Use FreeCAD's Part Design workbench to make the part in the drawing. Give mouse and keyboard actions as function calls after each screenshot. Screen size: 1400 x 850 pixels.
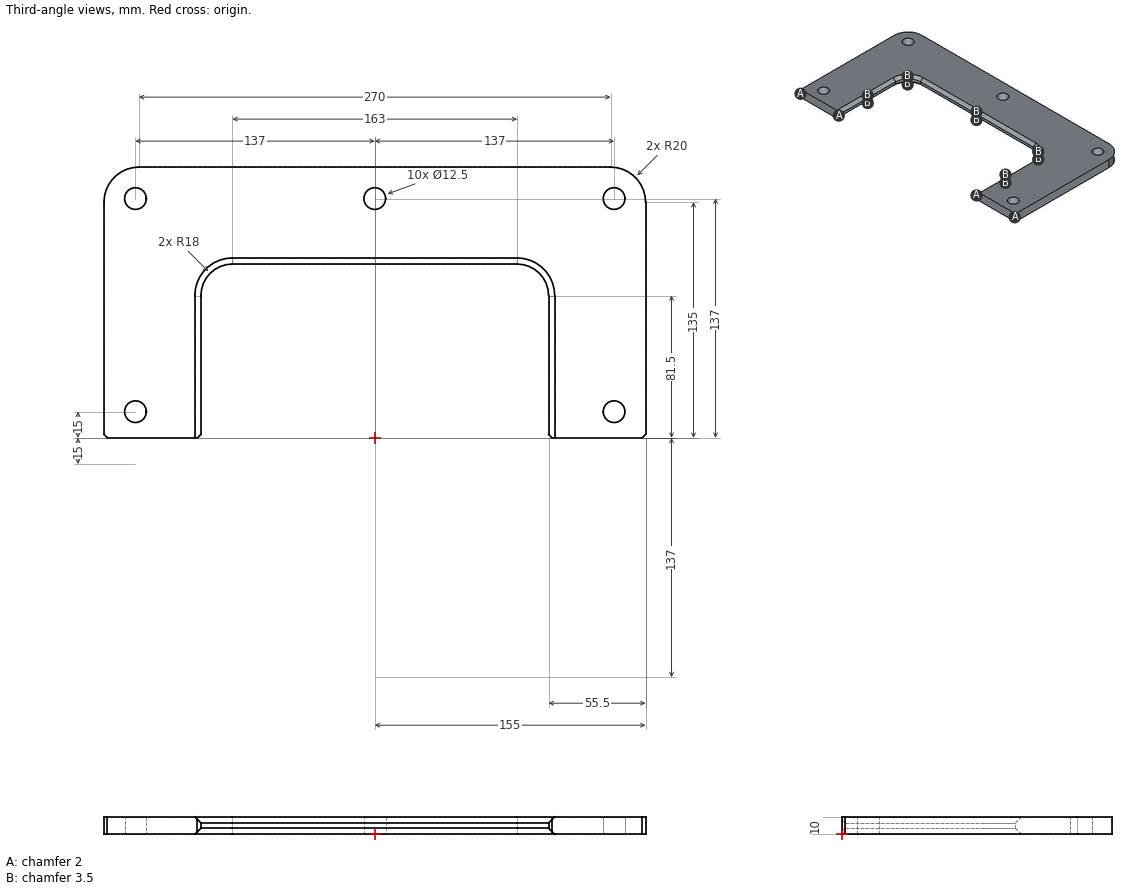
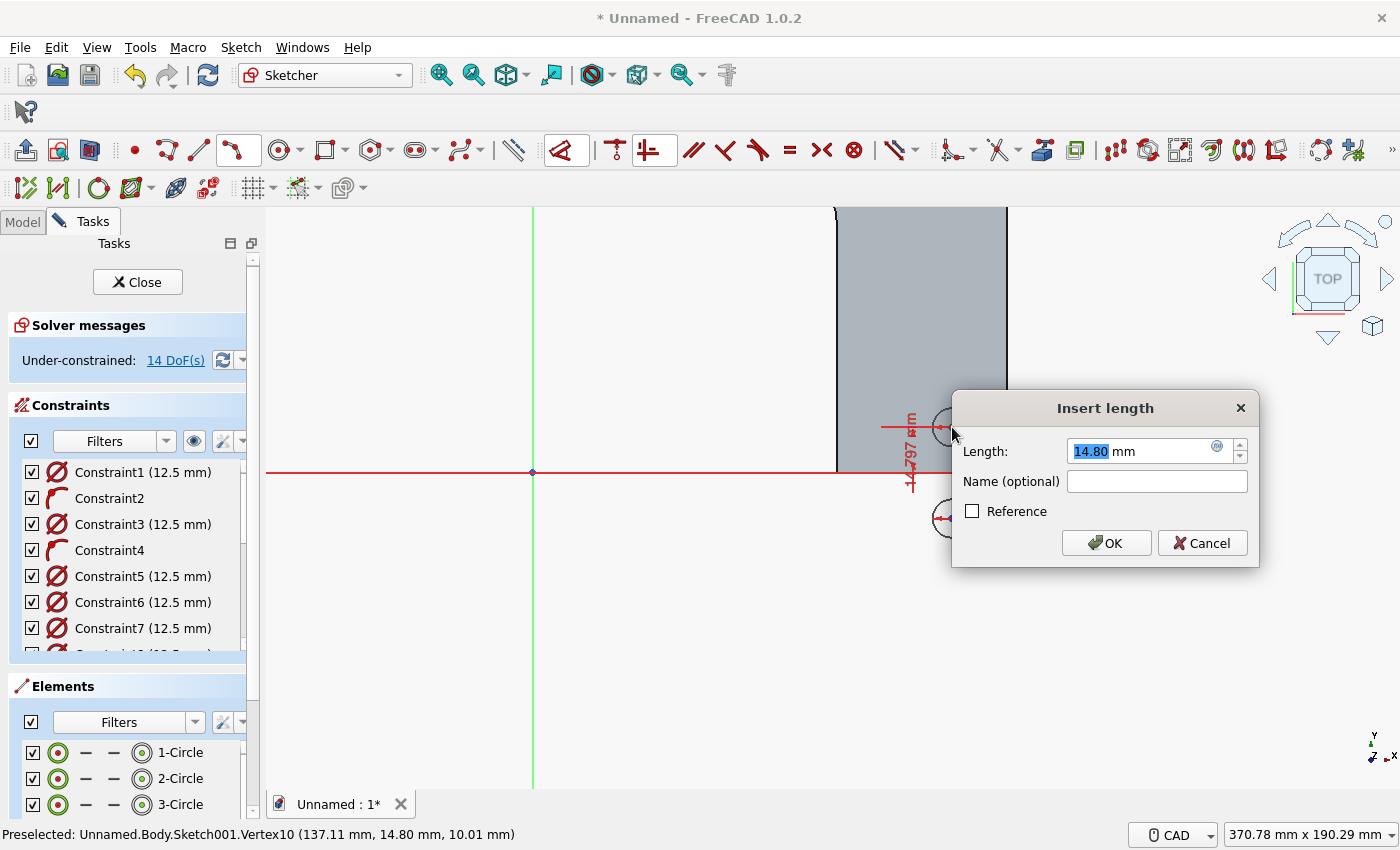
text(15)
key(Return)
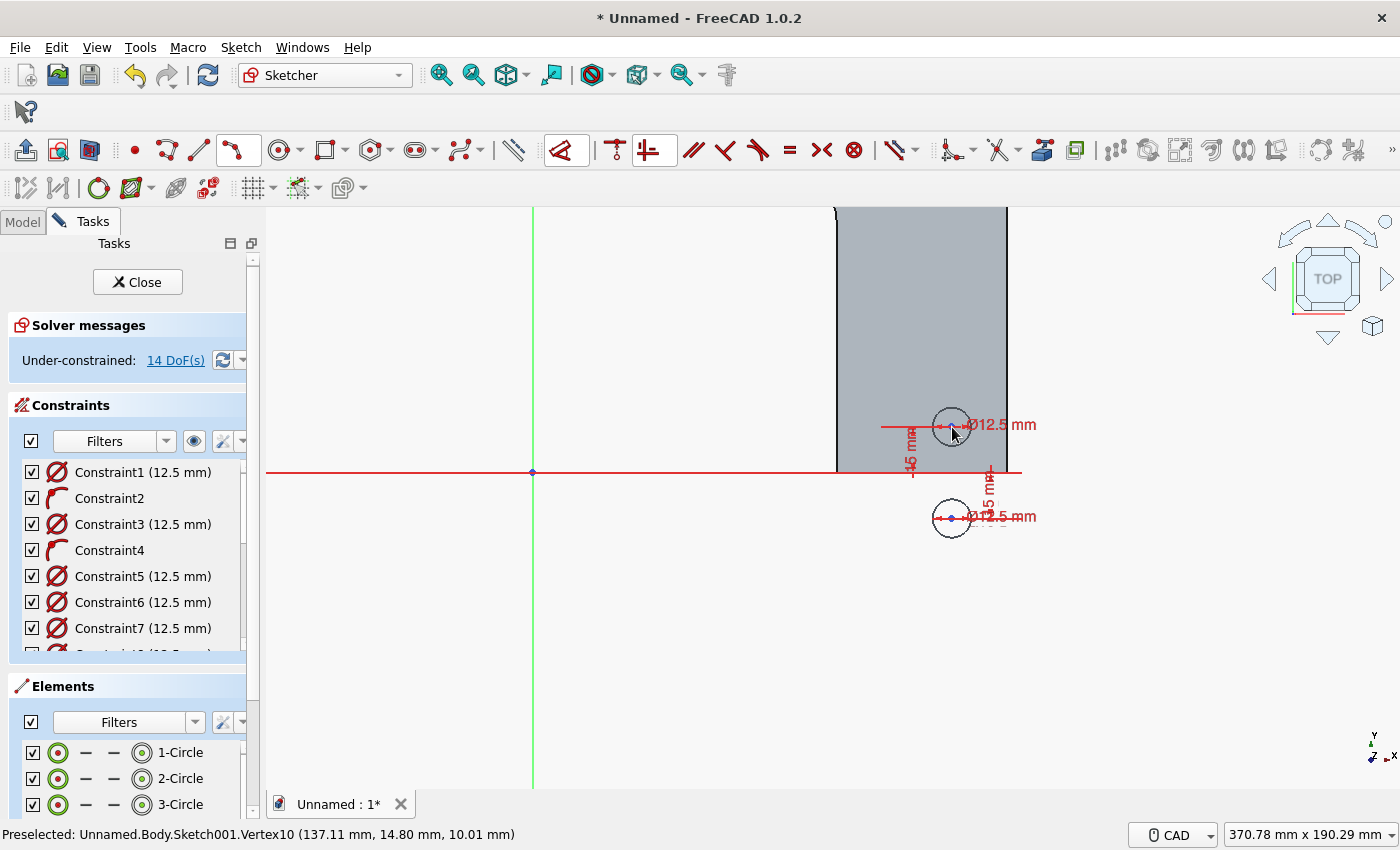
scroll(954, 519, down, 4)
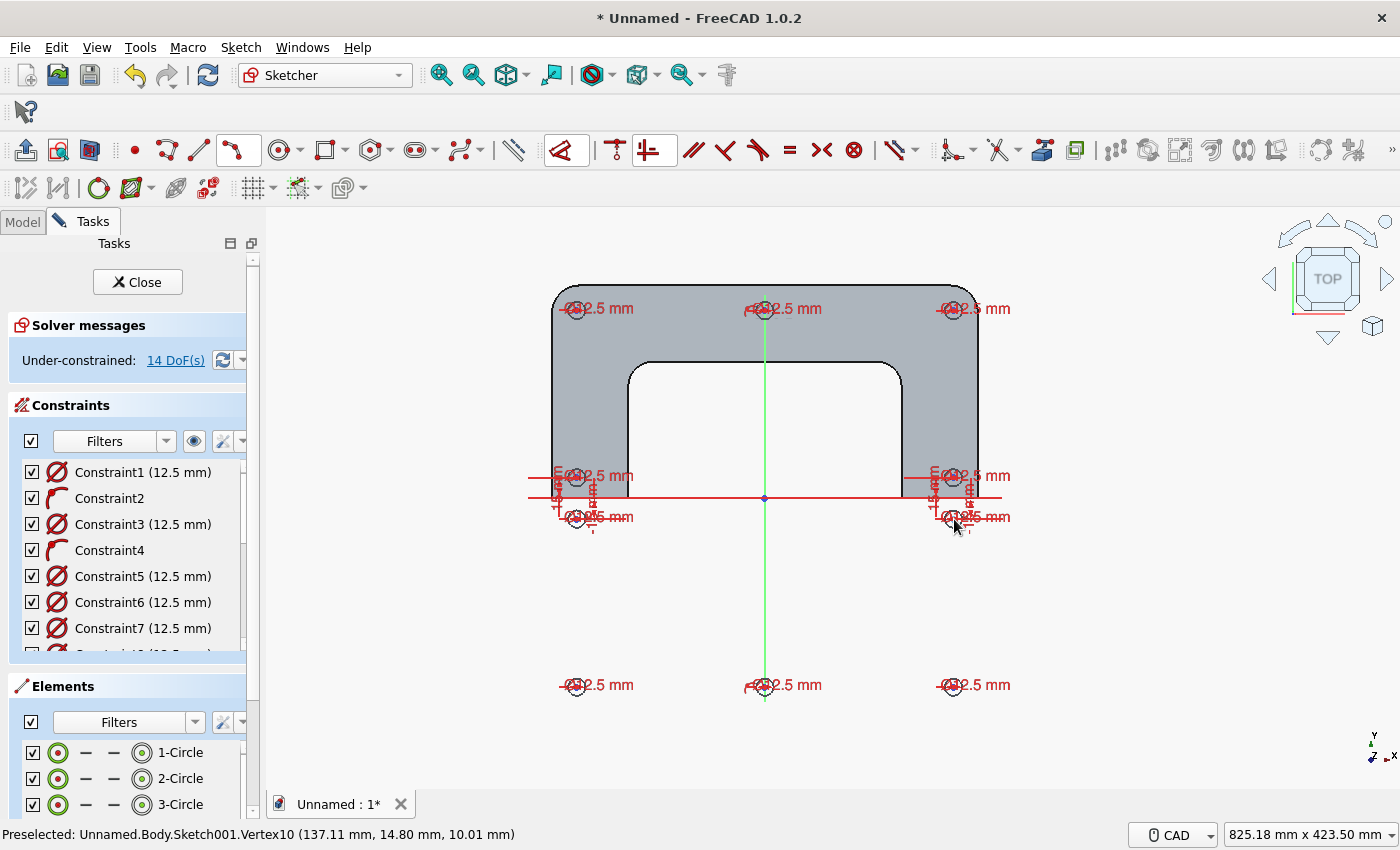
click(765, 311)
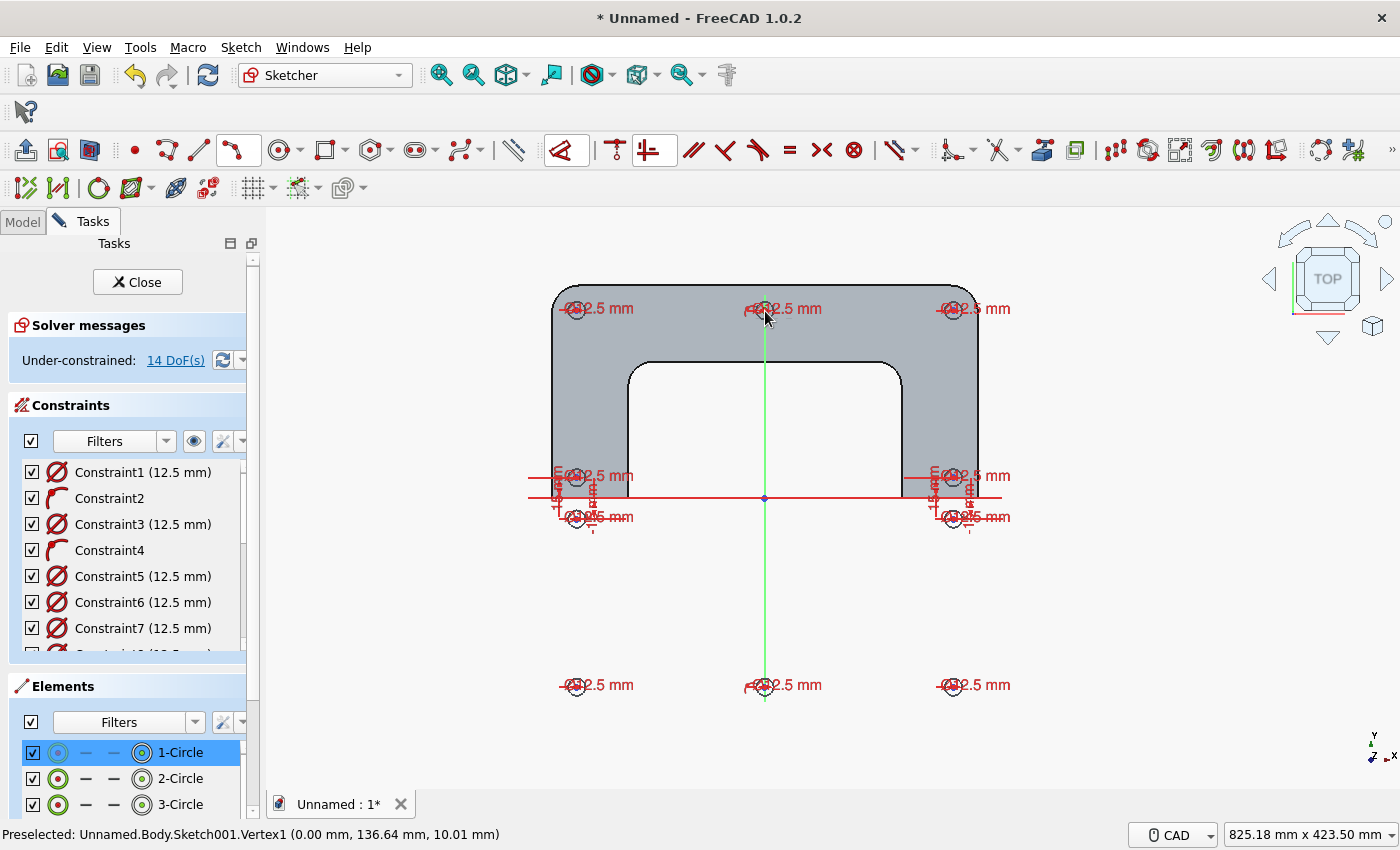
key(i)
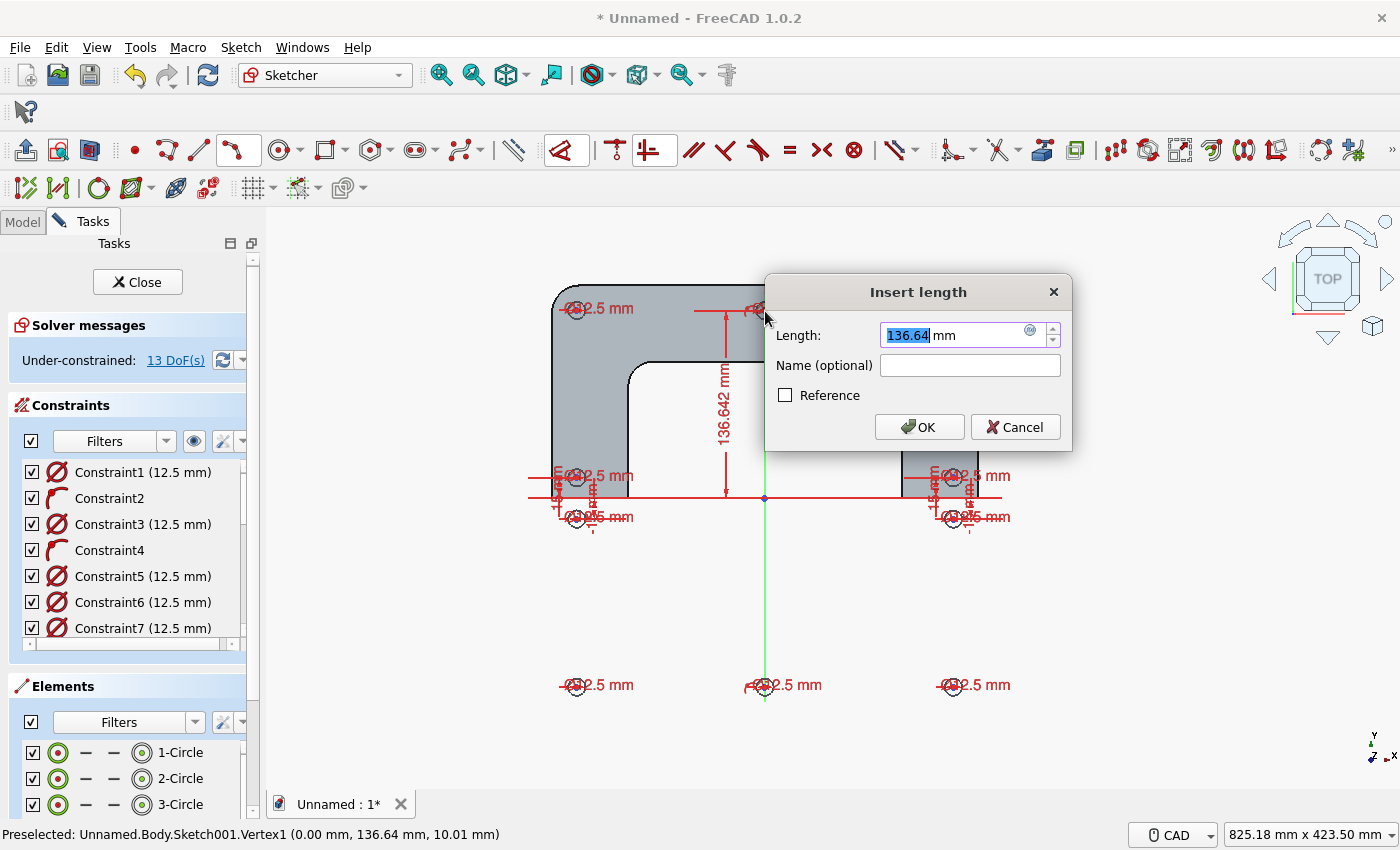
text(137)
key(Return)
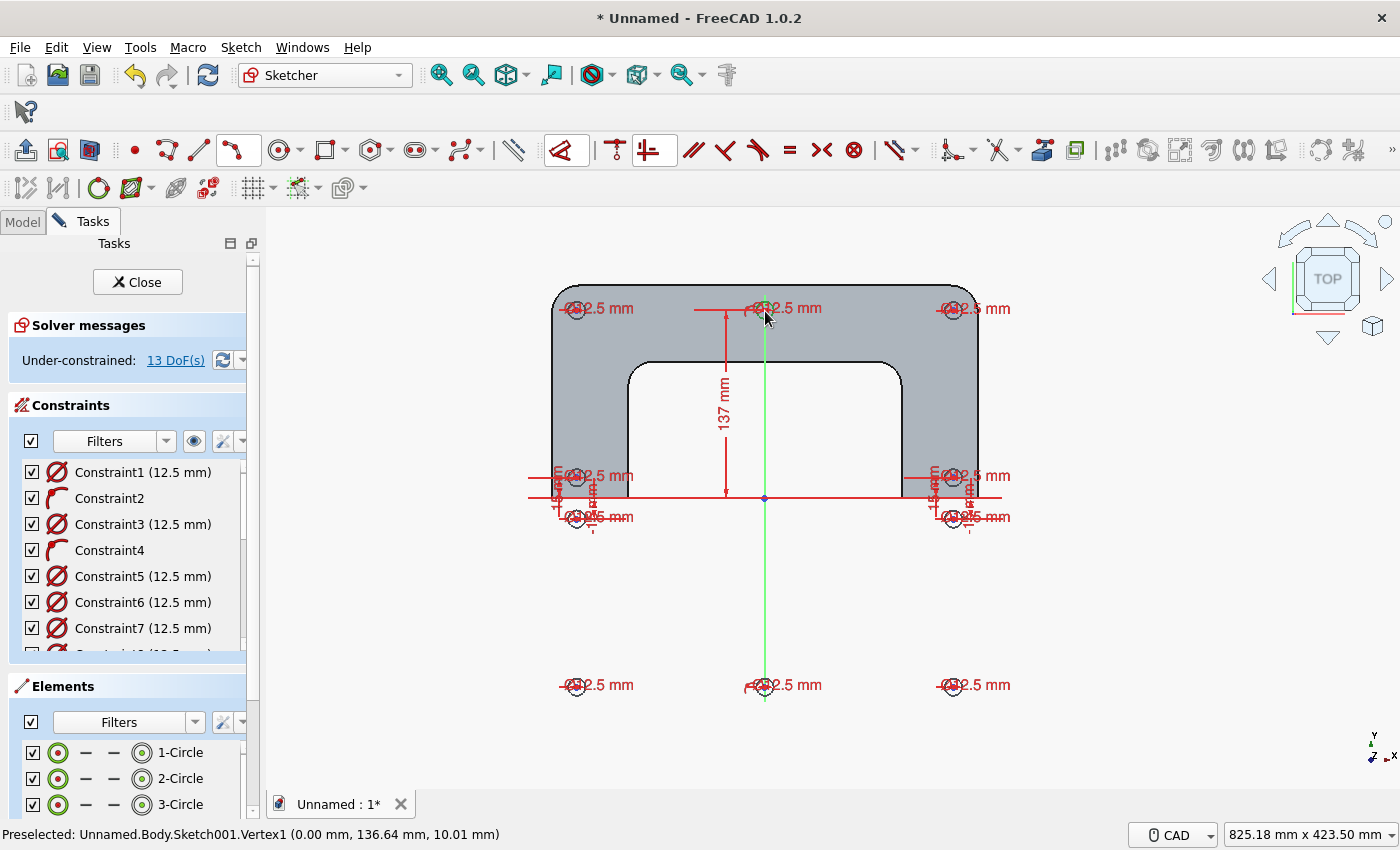
click(765, 687)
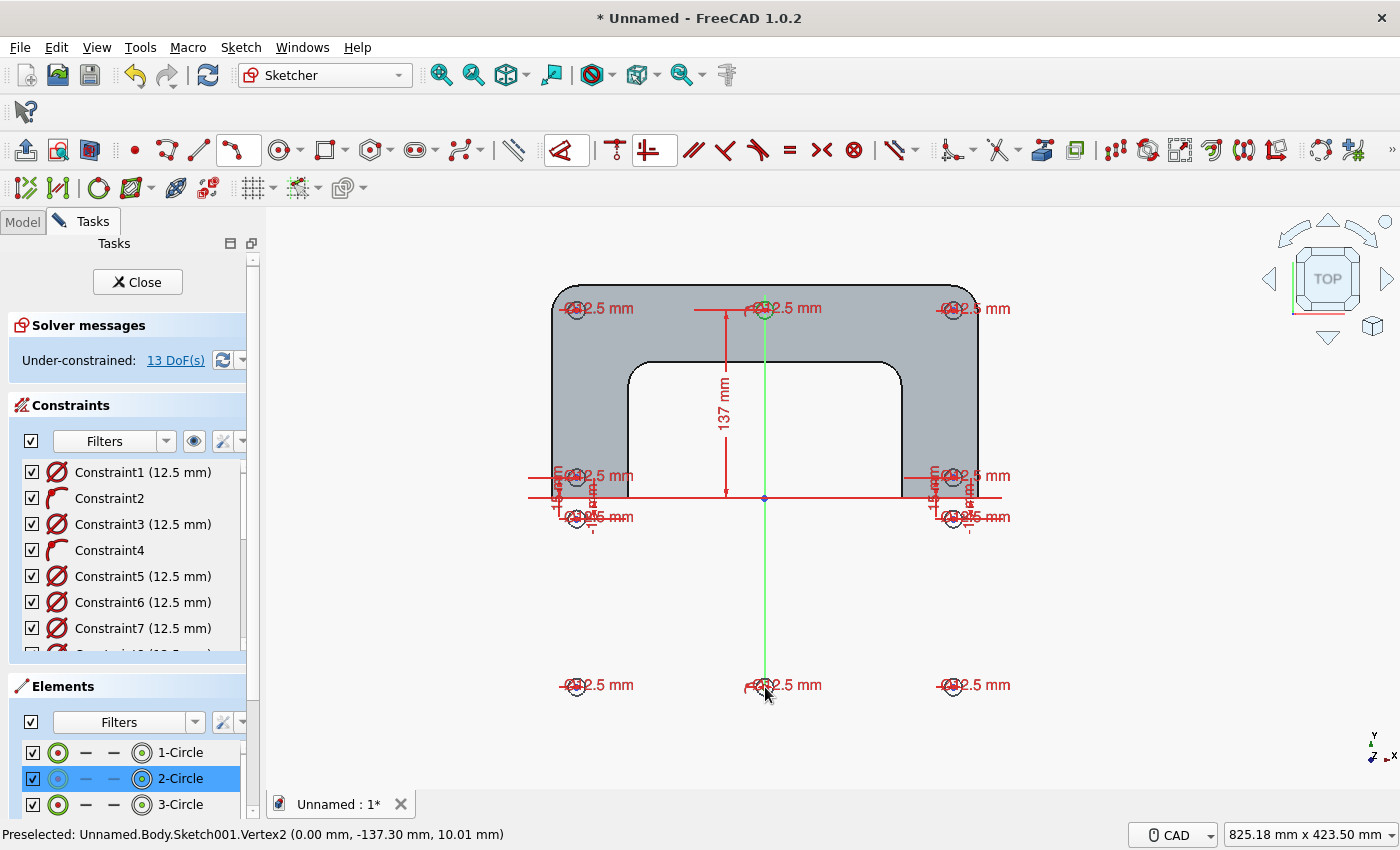
key(i)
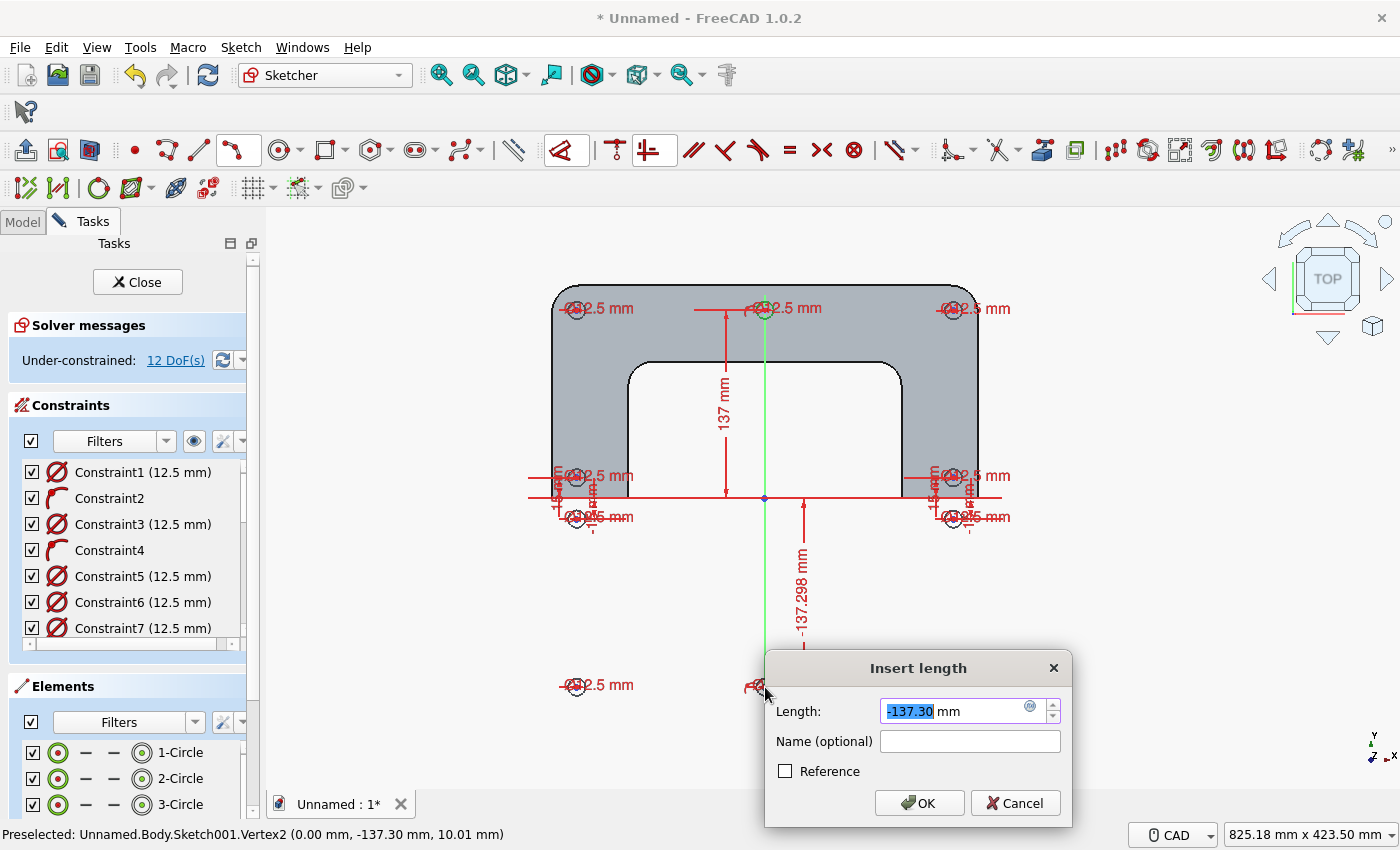
text(-137)
key(Return)